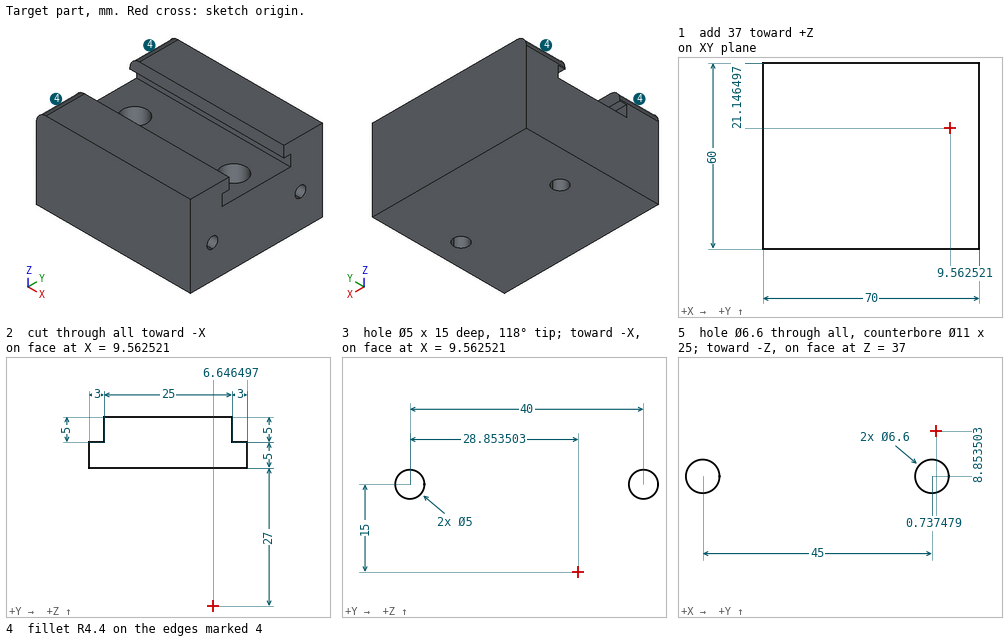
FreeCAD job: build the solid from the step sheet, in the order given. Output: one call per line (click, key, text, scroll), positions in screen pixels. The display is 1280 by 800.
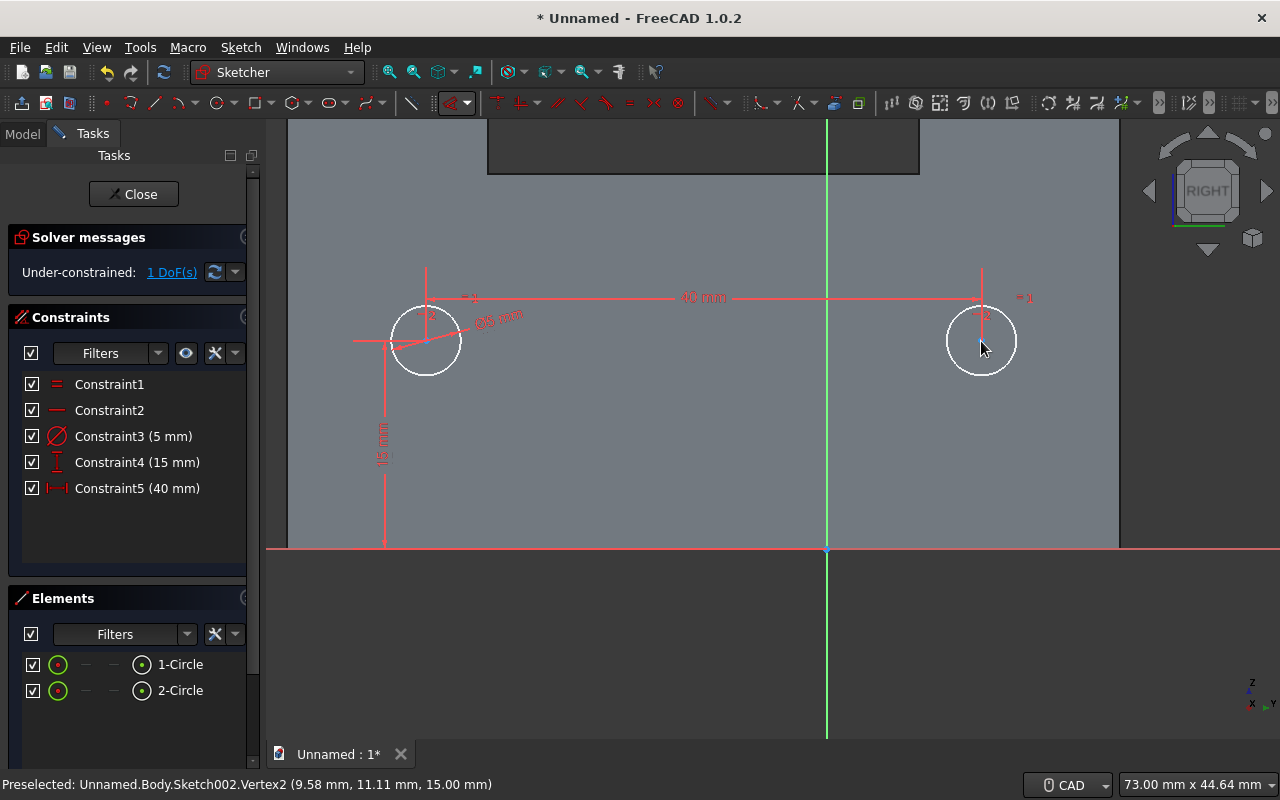
click(426, 341)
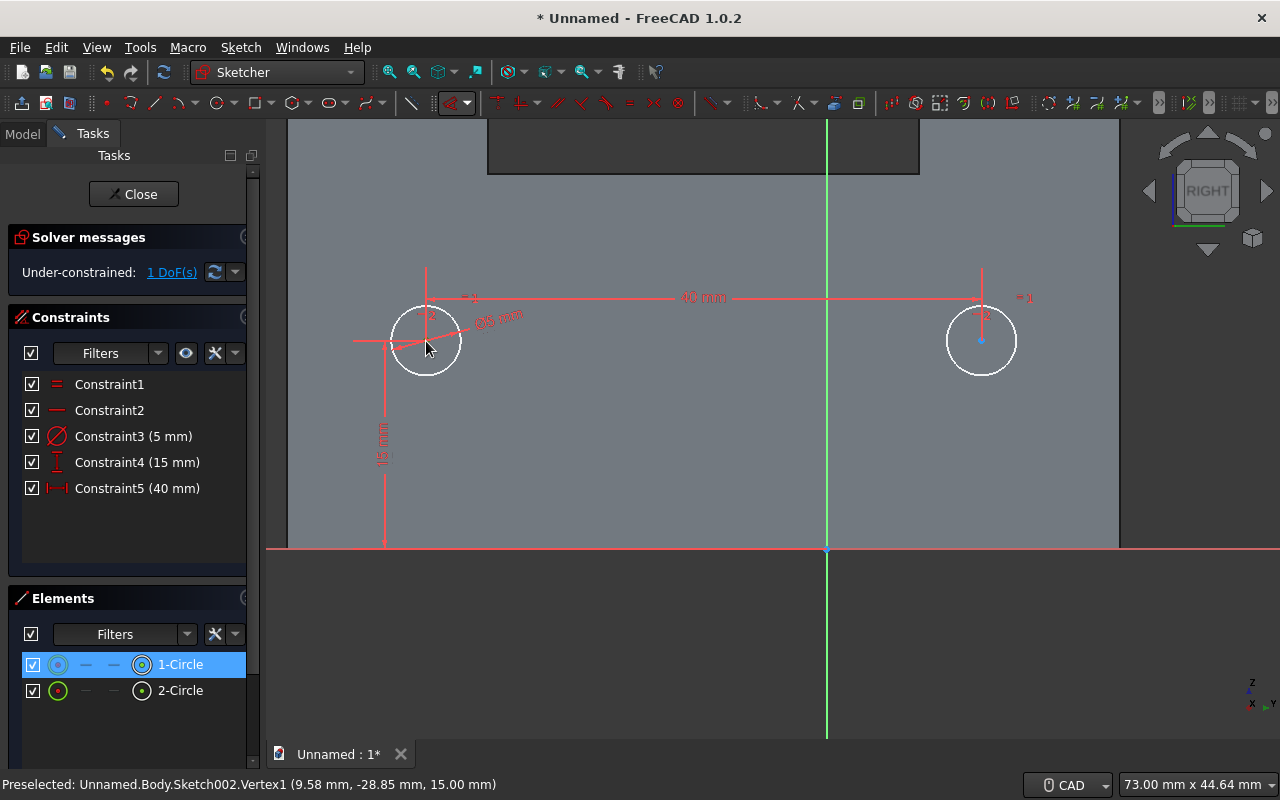
click(470, 104)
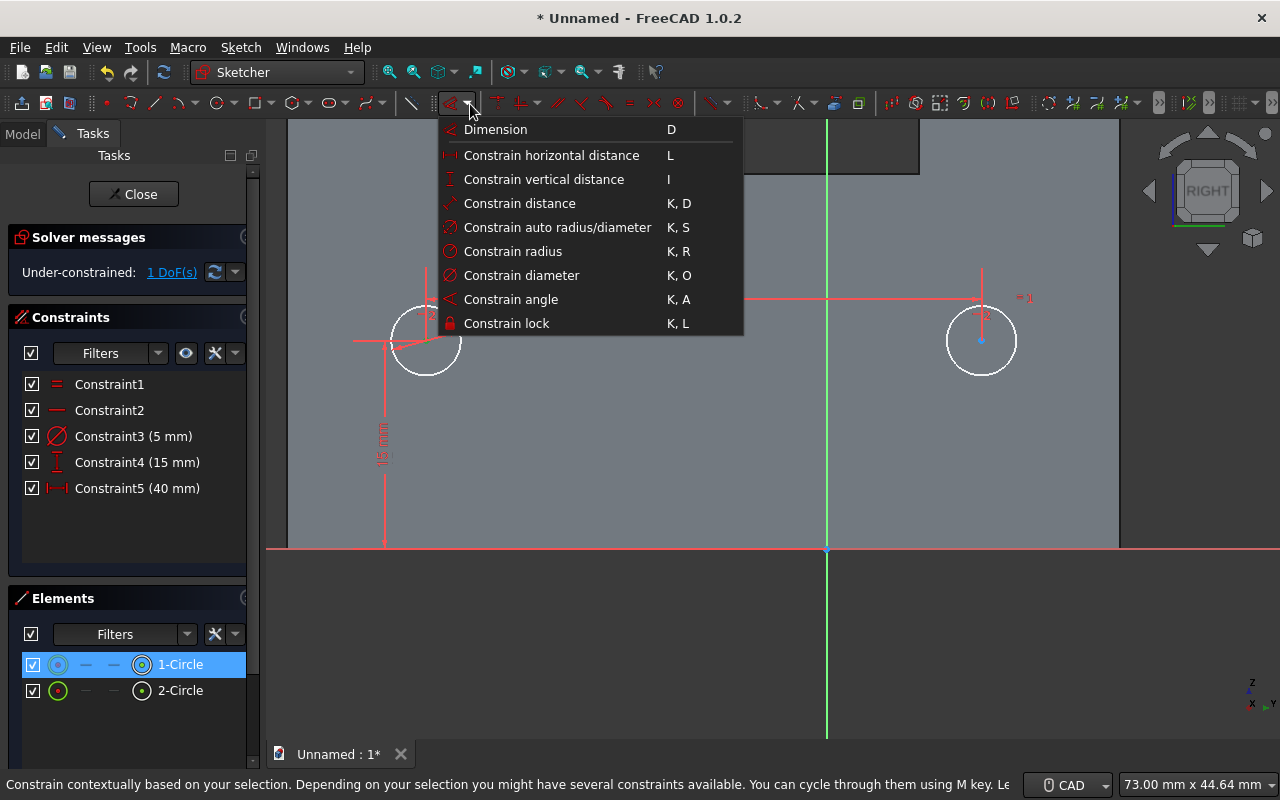
click(591, 155)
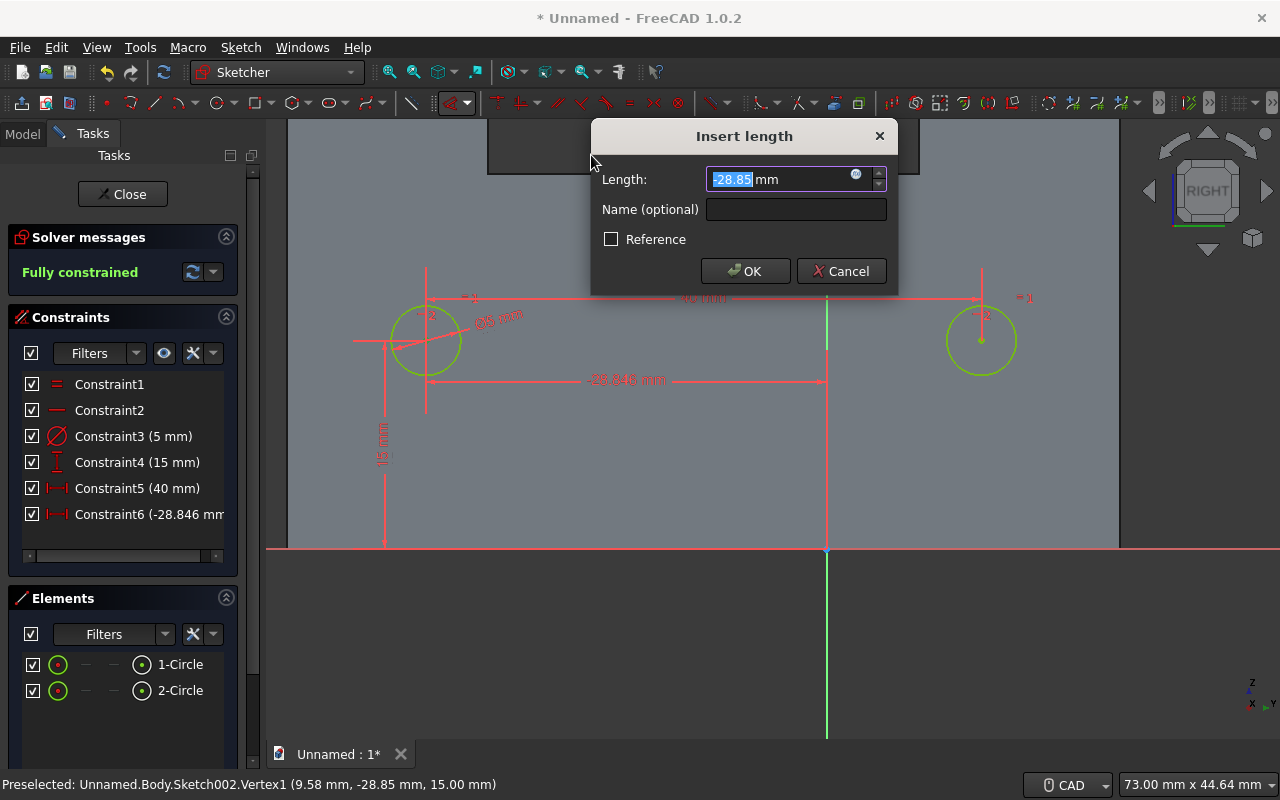
text(-28.853503)
key(Return)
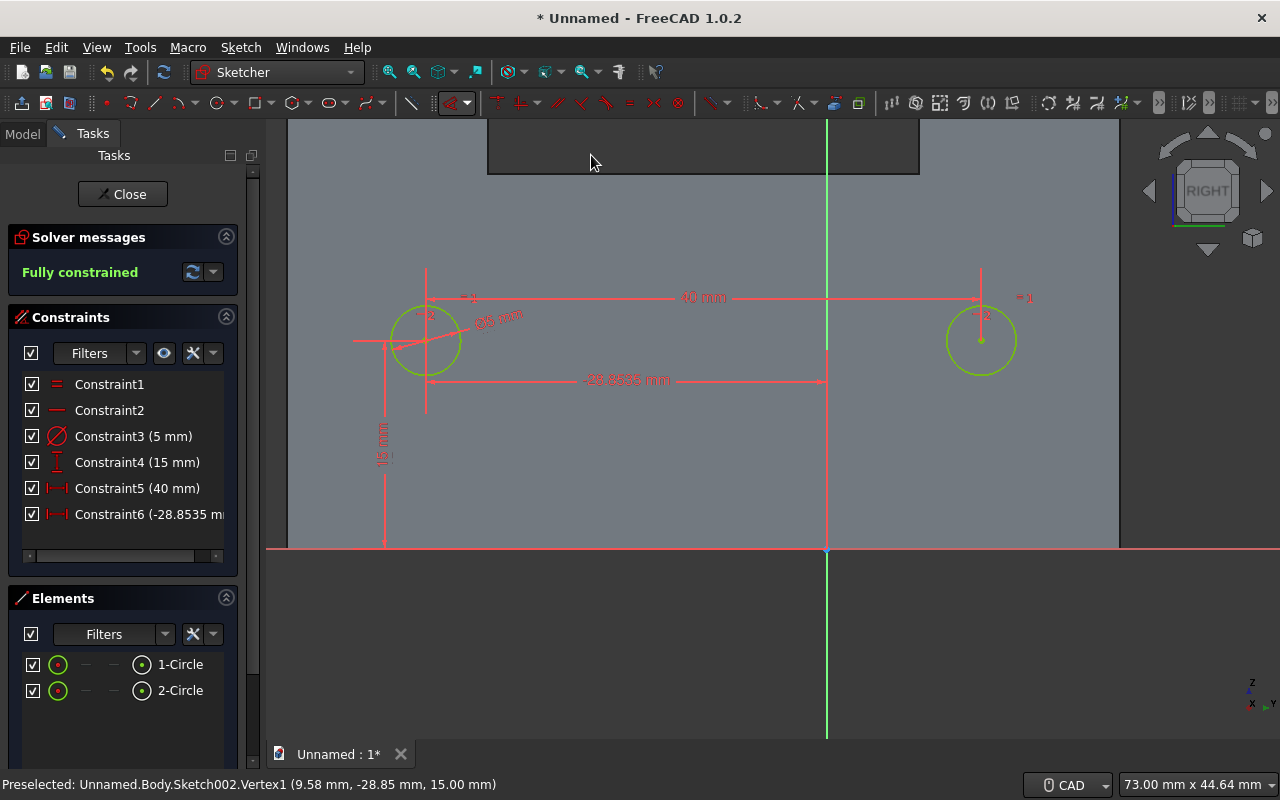
click(123, 194)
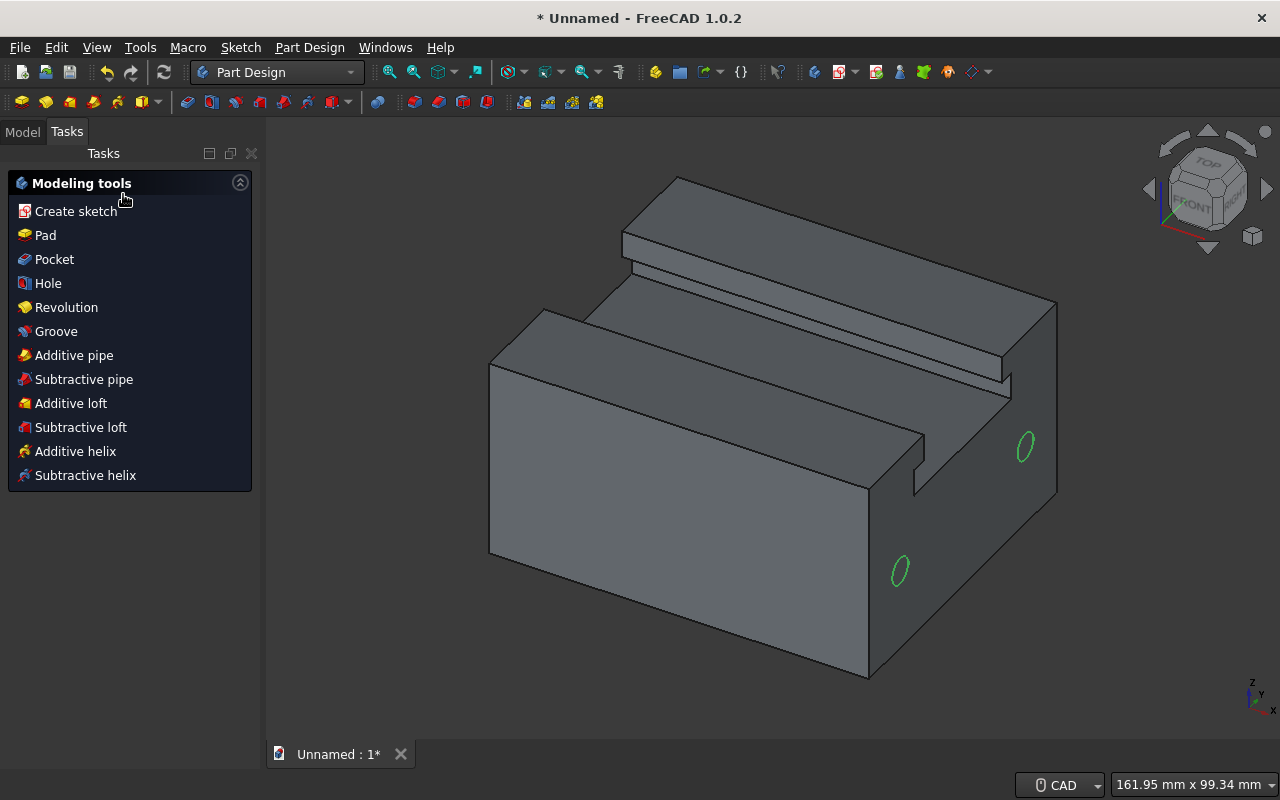
click(212, 102)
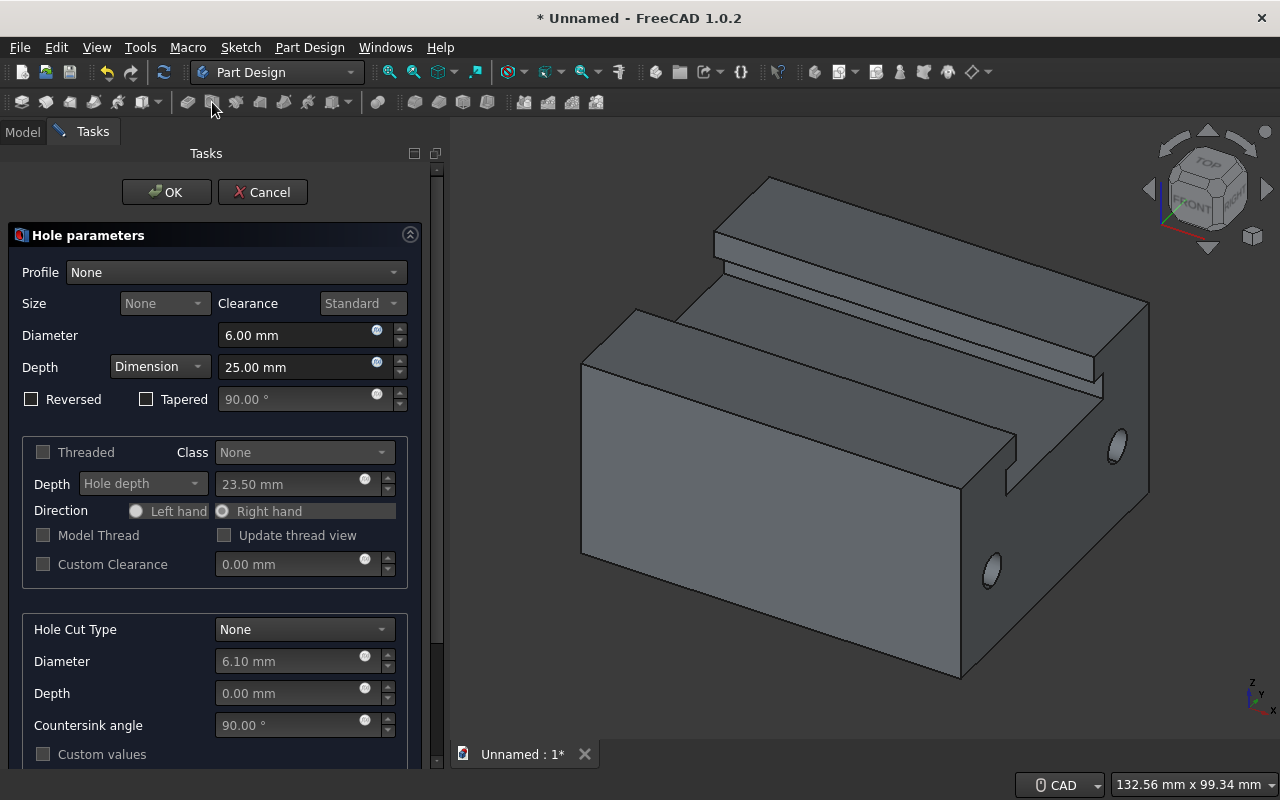
triple_click(305, 335)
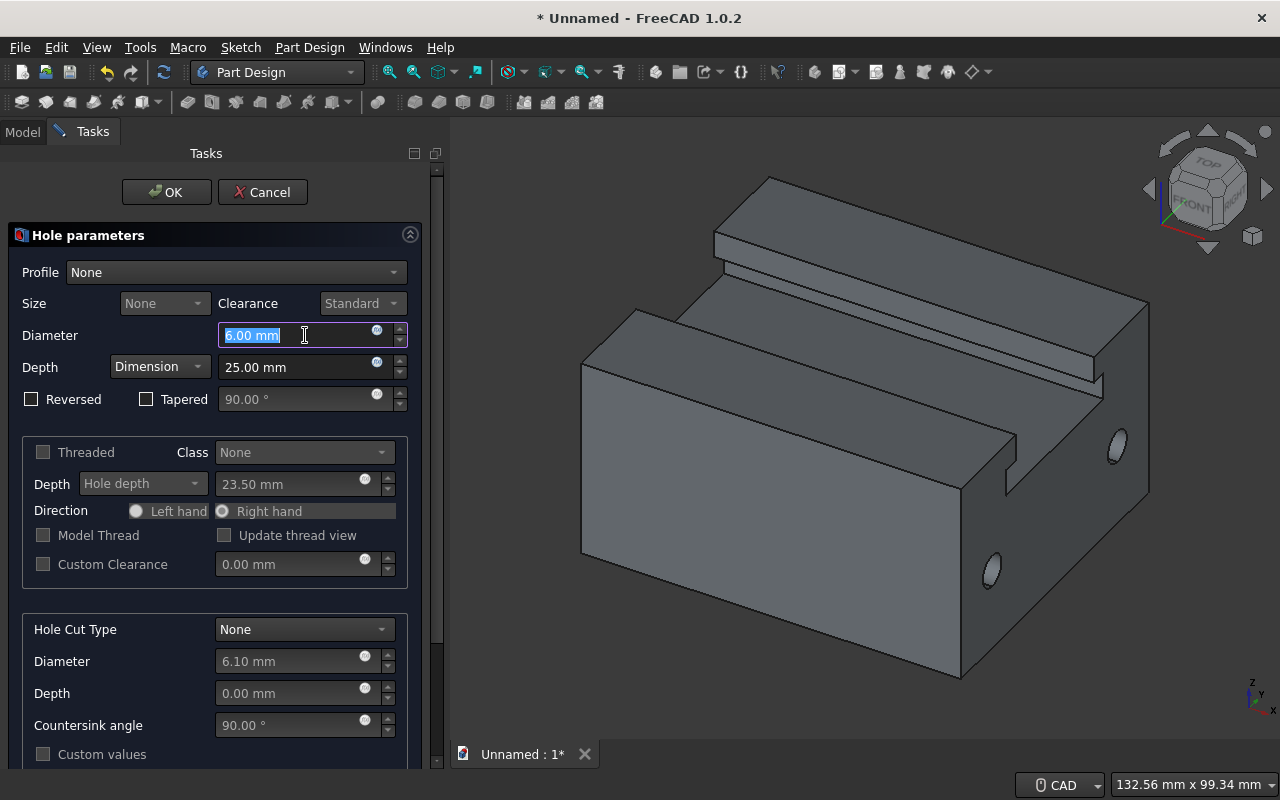
text(5)
key(Tab)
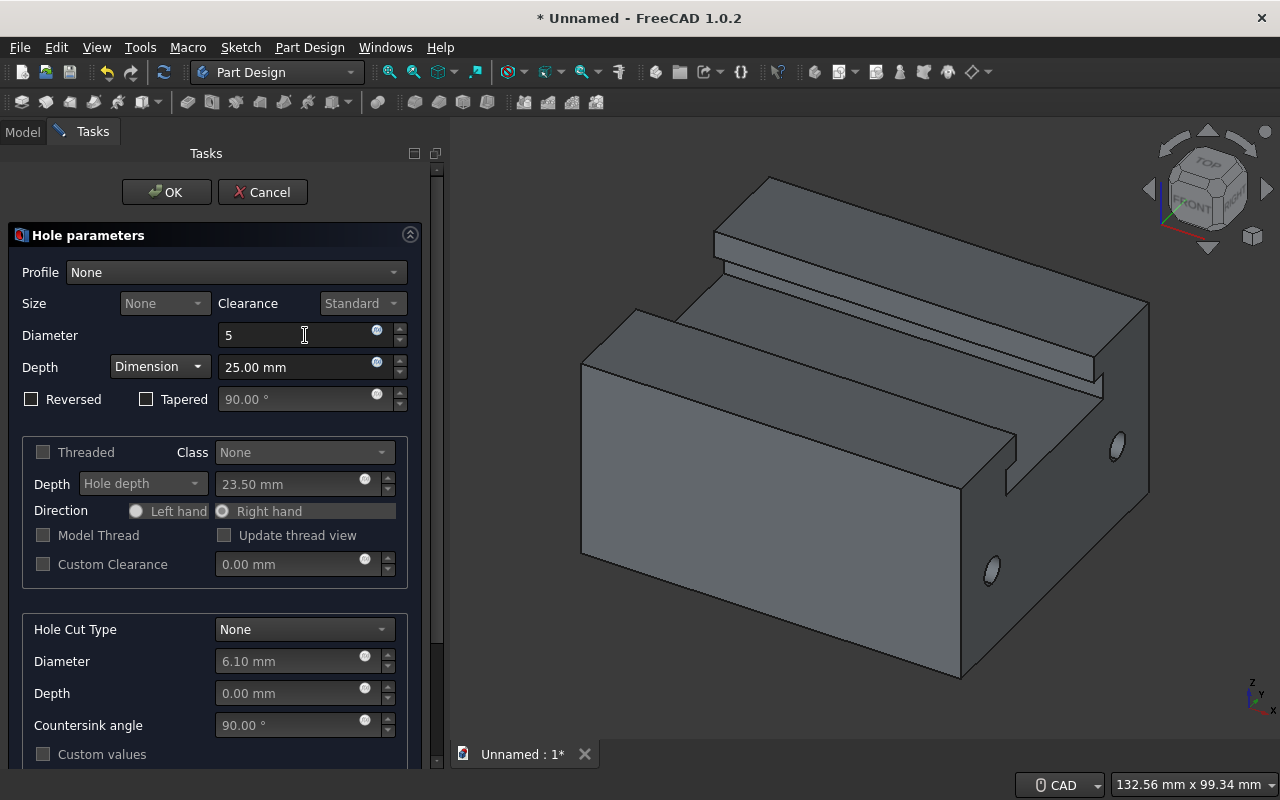
triple_click(305, 367)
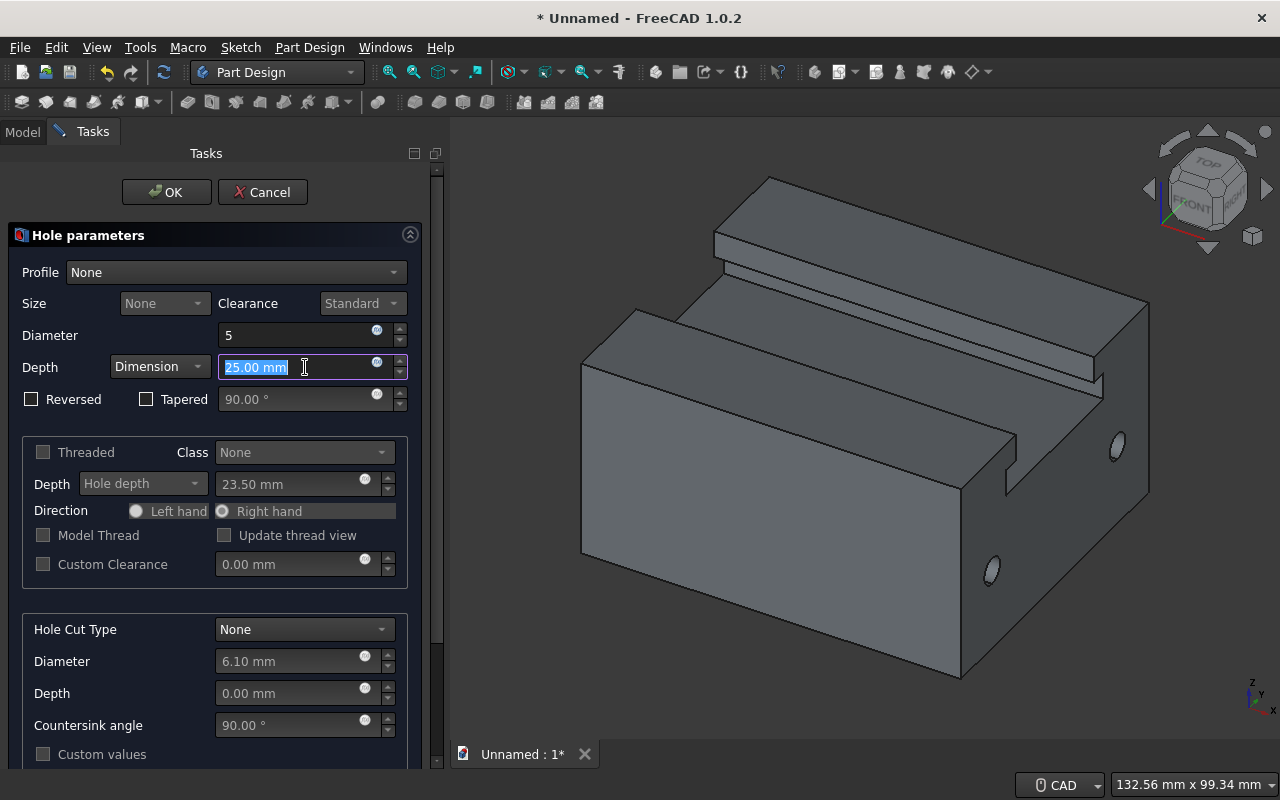
text(15)
key(Tab)